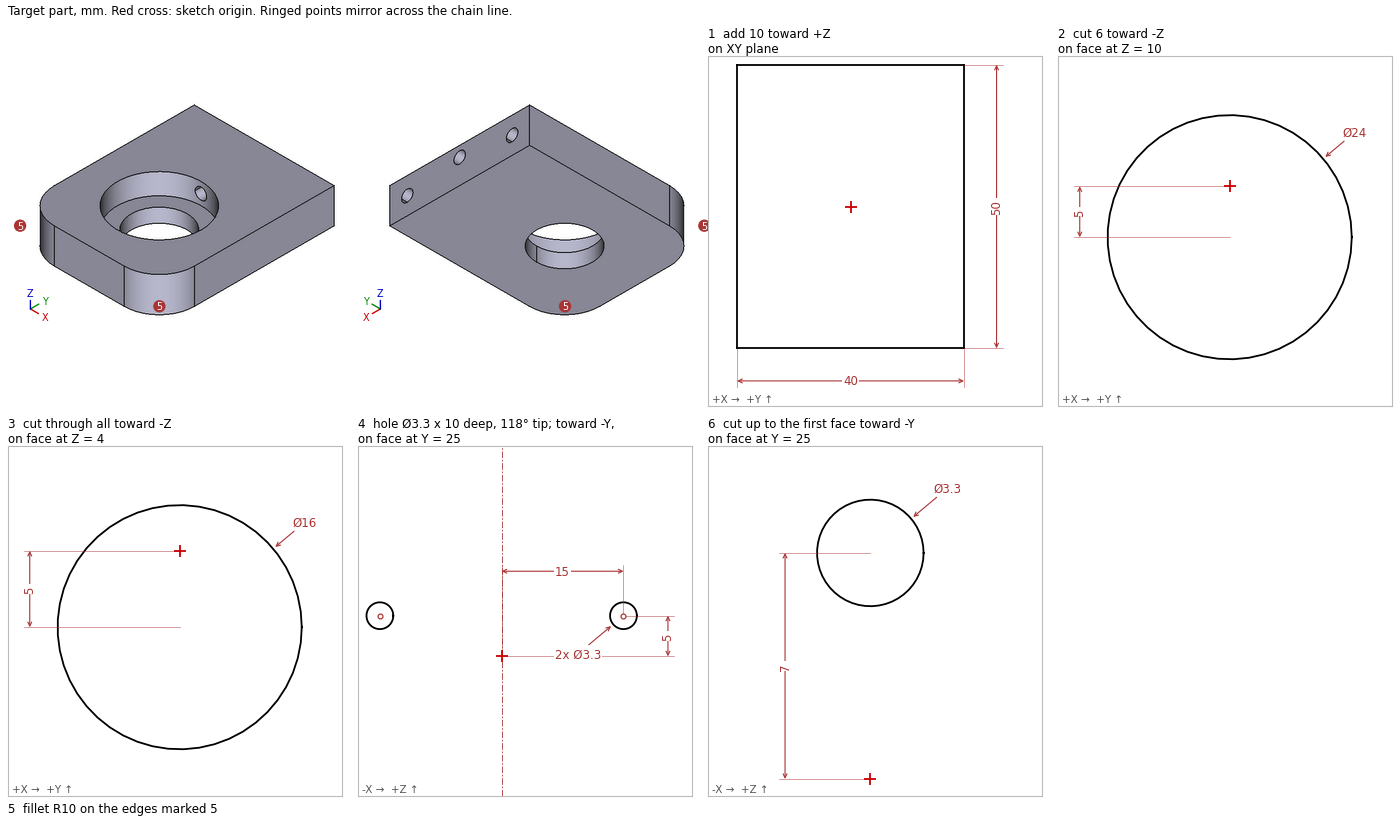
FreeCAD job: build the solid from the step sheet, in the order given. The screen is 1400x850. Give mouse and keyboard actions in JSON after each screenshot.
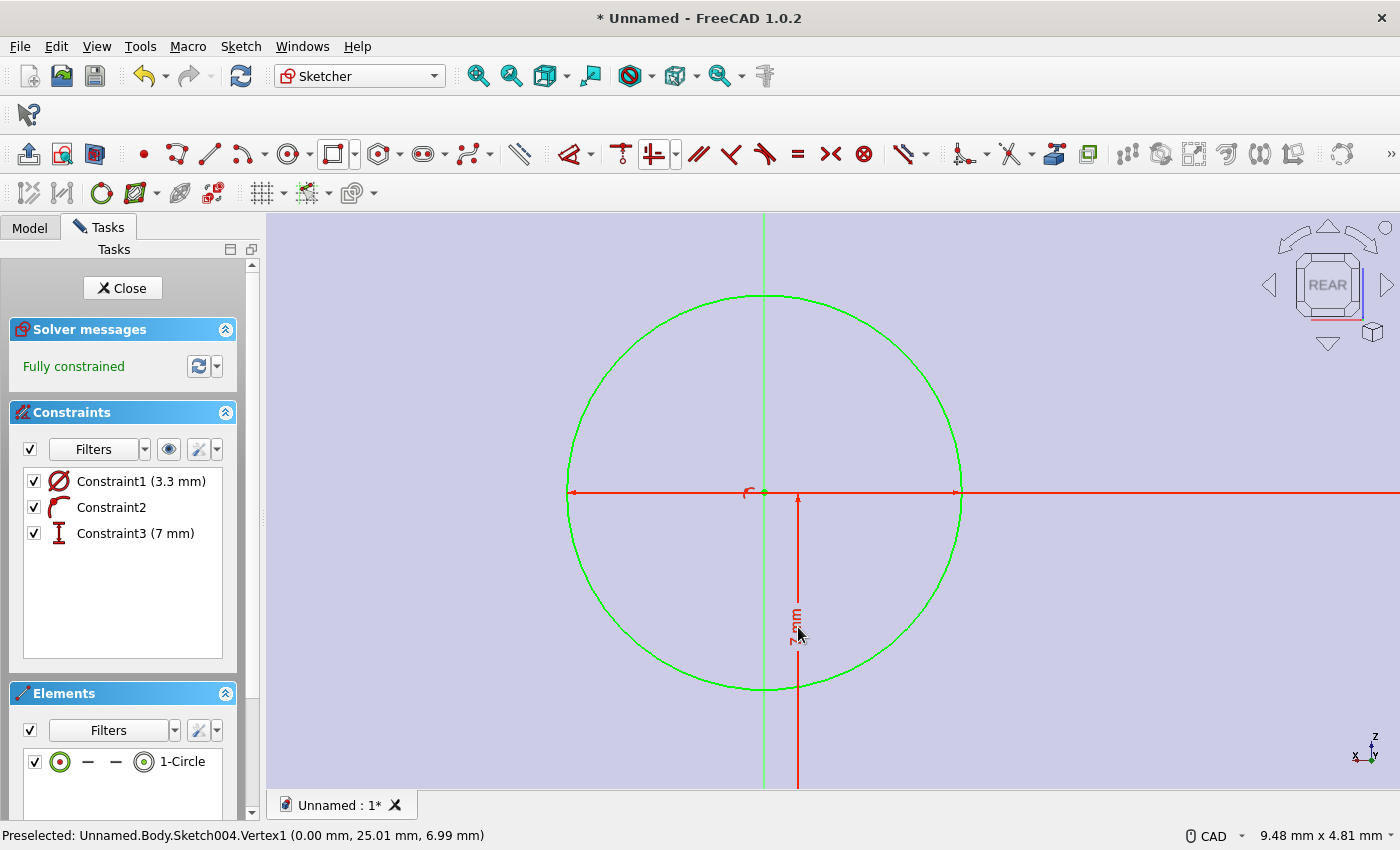
{"action": "left_click", "coordinate": [123, 288]}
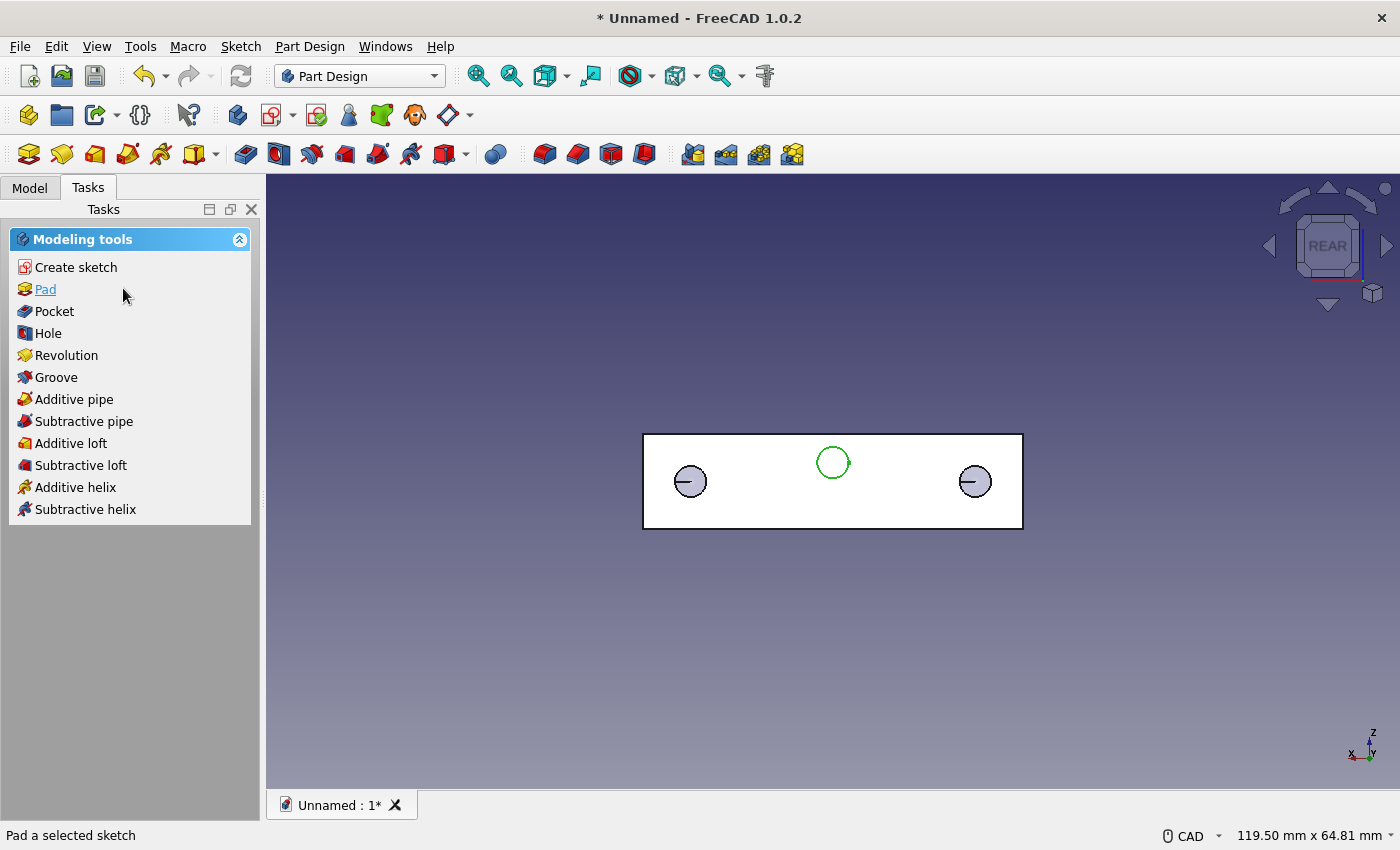
{"action": "left_click", "coordinate": [246, 154]}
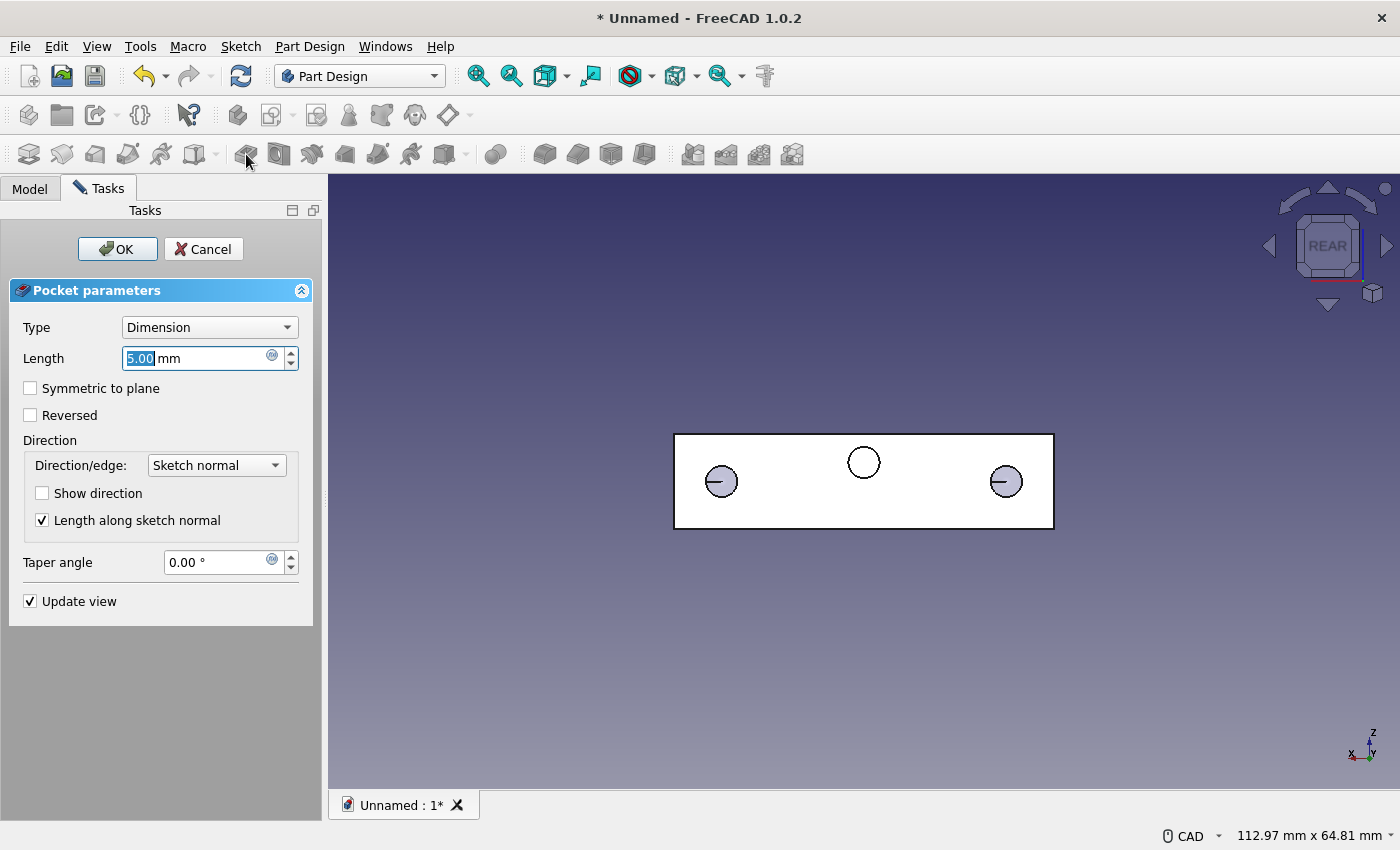
{"action": "left_click", "coordinate": [210, 328]}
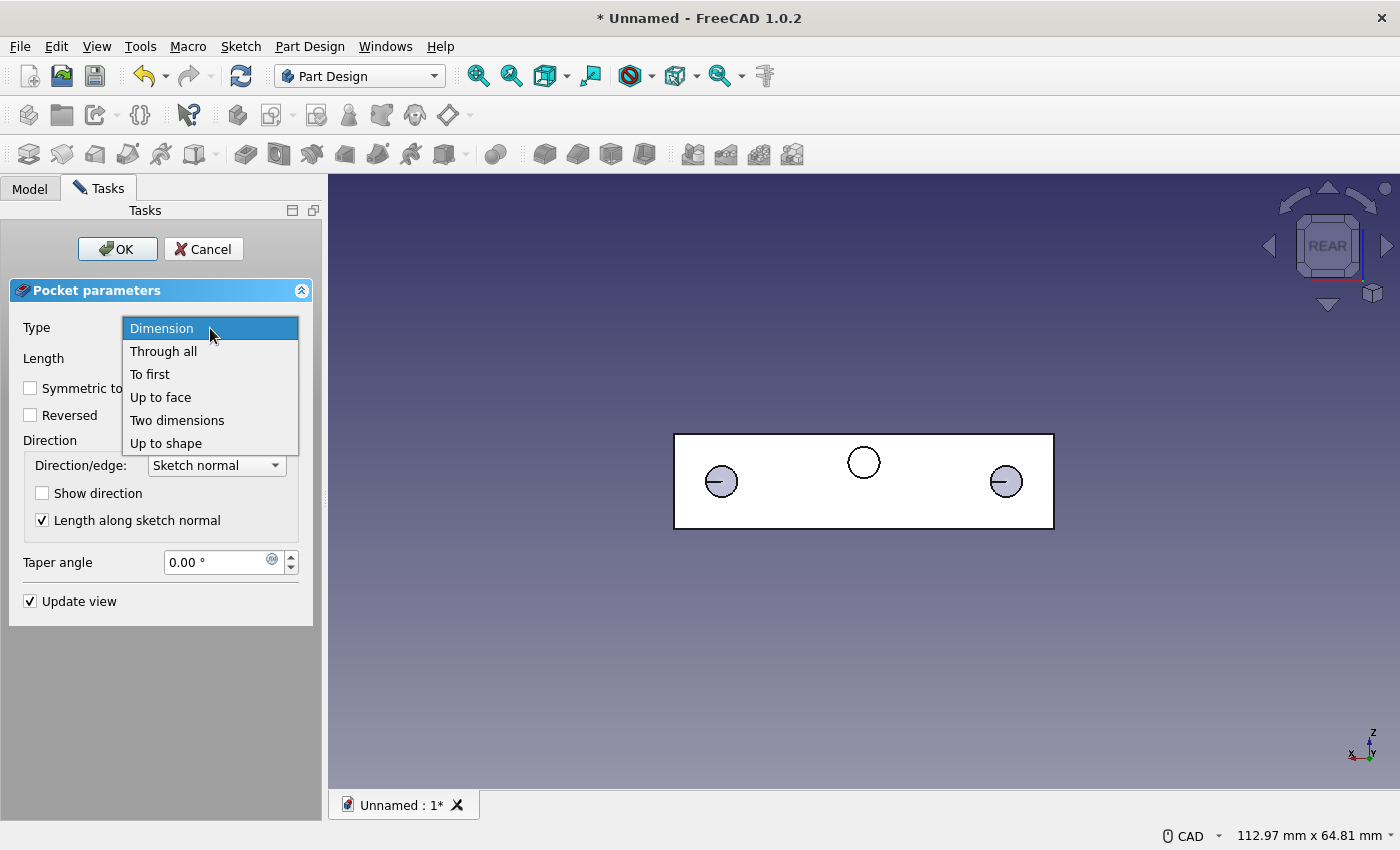
{"action": "left_click", "coordinate": [208, 374]}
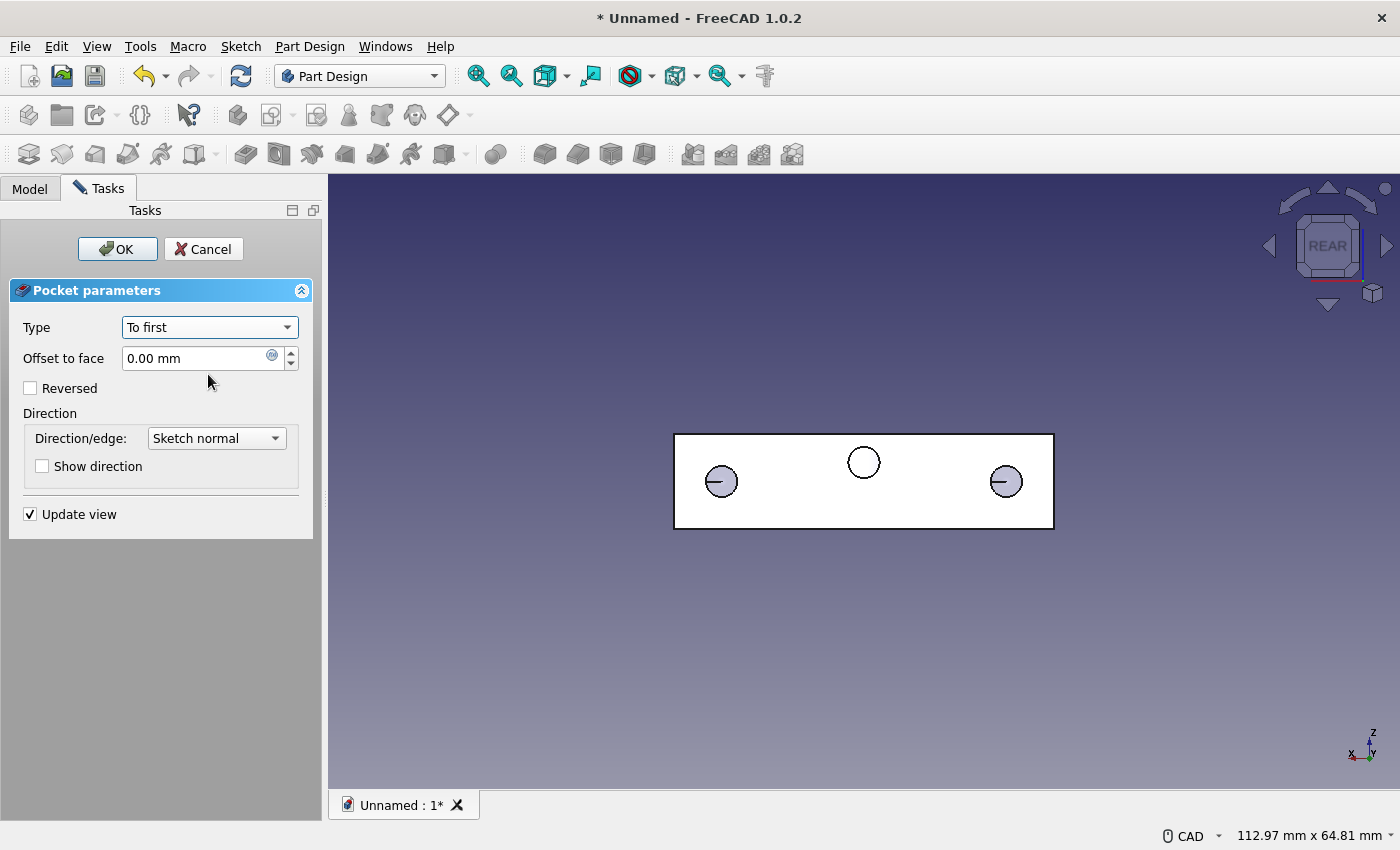
{"action": "left_click", "coordinate": [118, 249]}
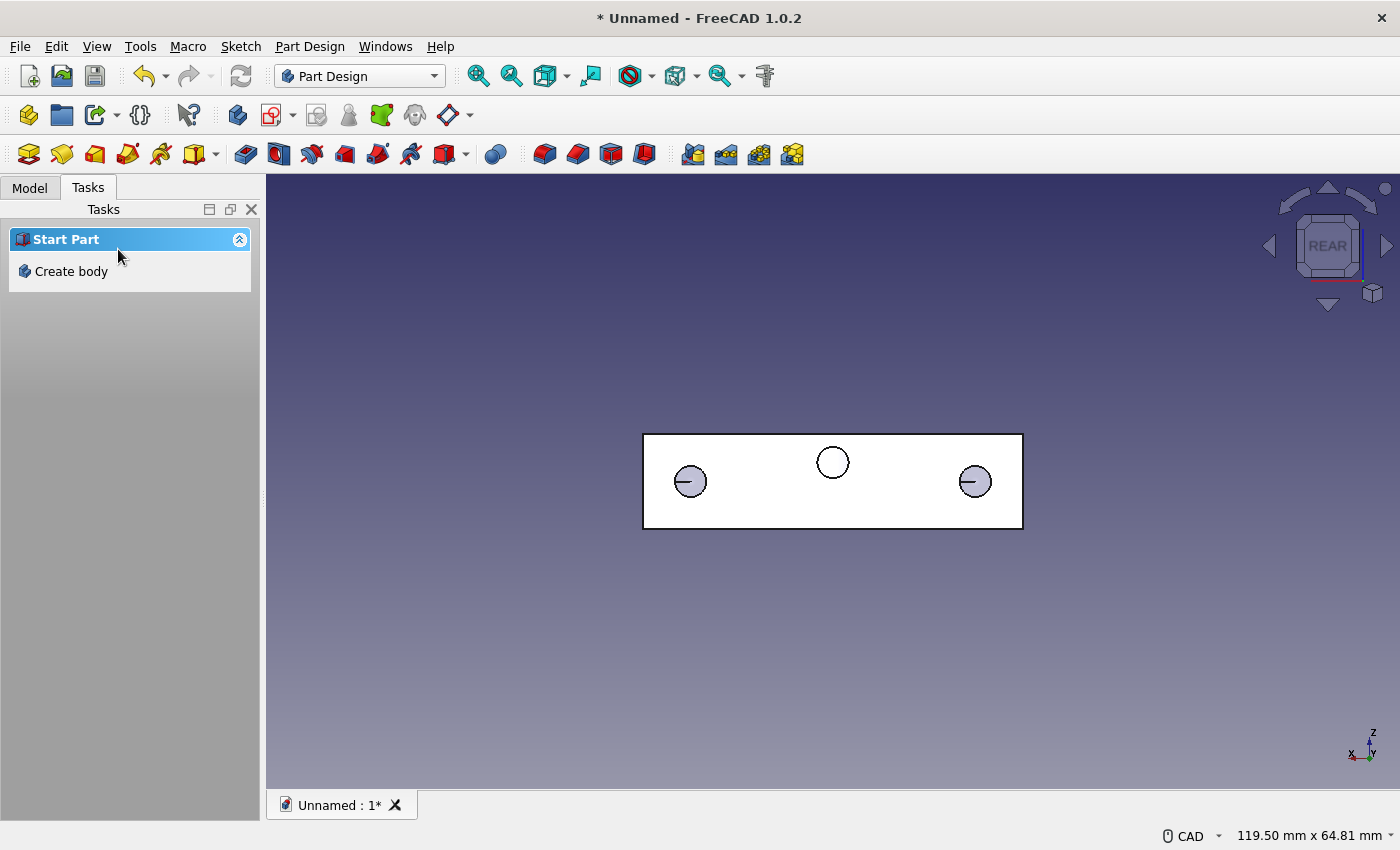
{"action": "key", "text": "0"}